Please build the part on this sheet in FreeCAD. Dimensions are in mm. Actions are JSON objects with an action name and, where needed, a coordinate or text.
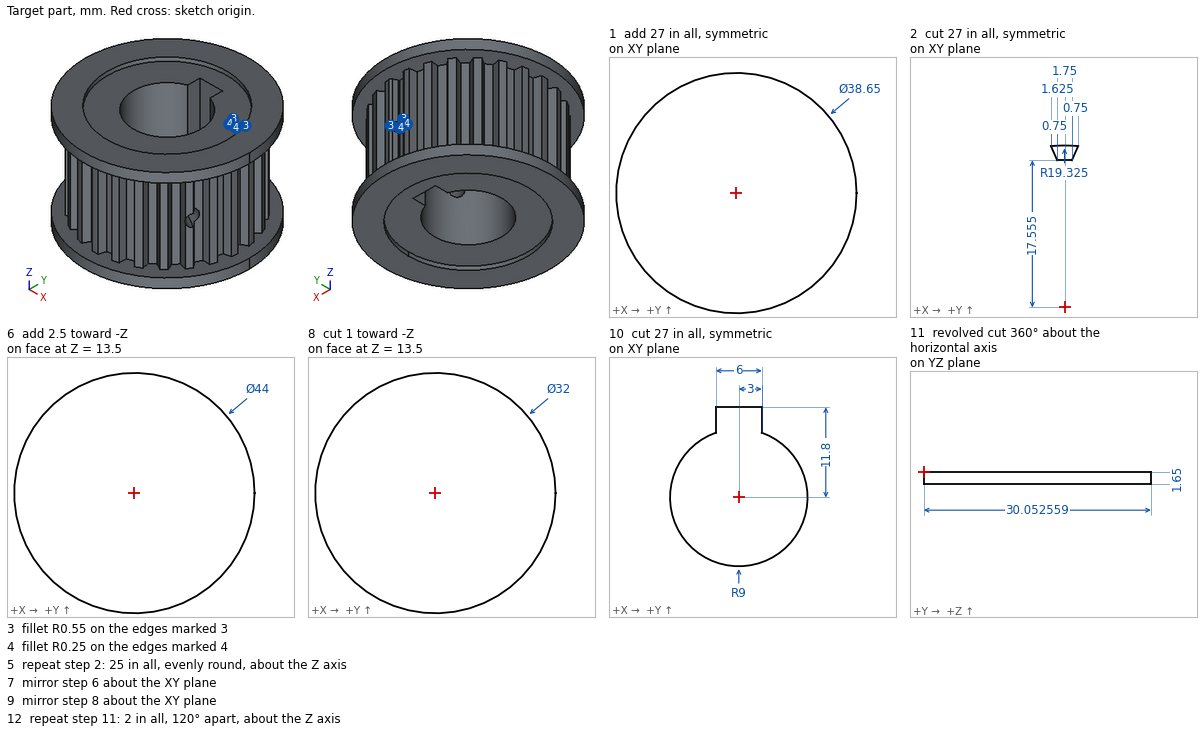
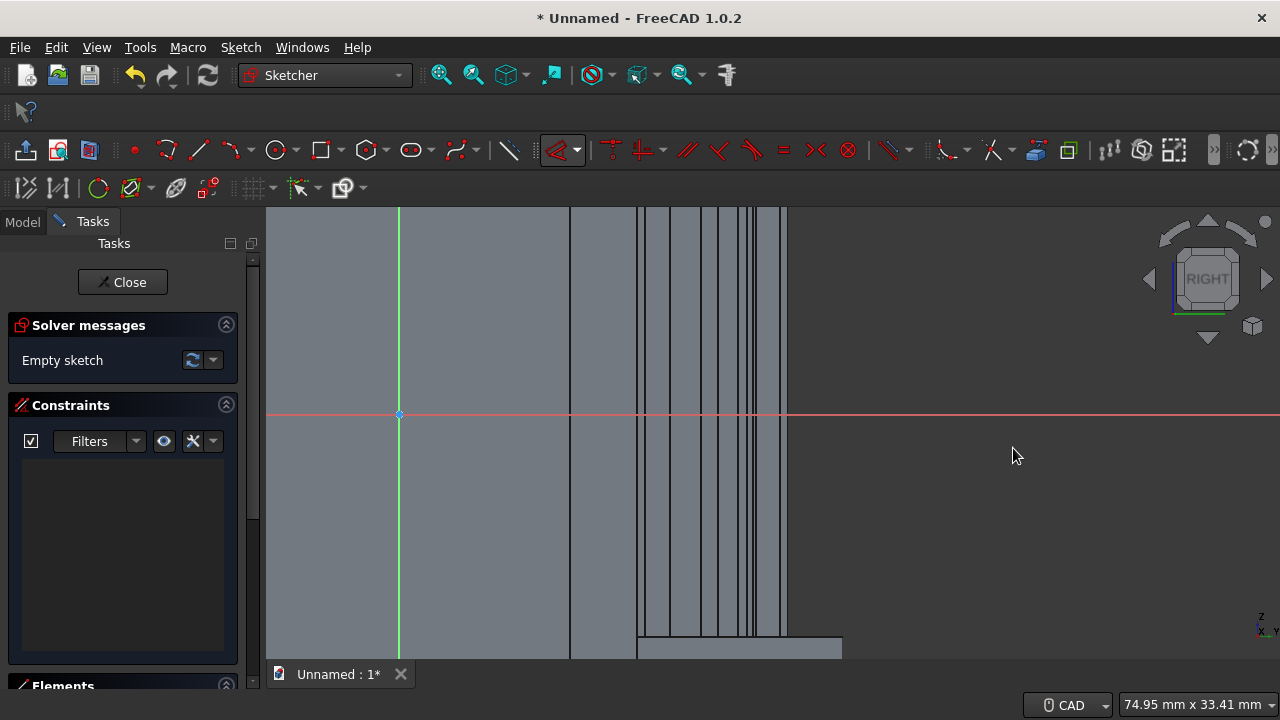
{"action": "left_click", "coordinate": [322, 150]}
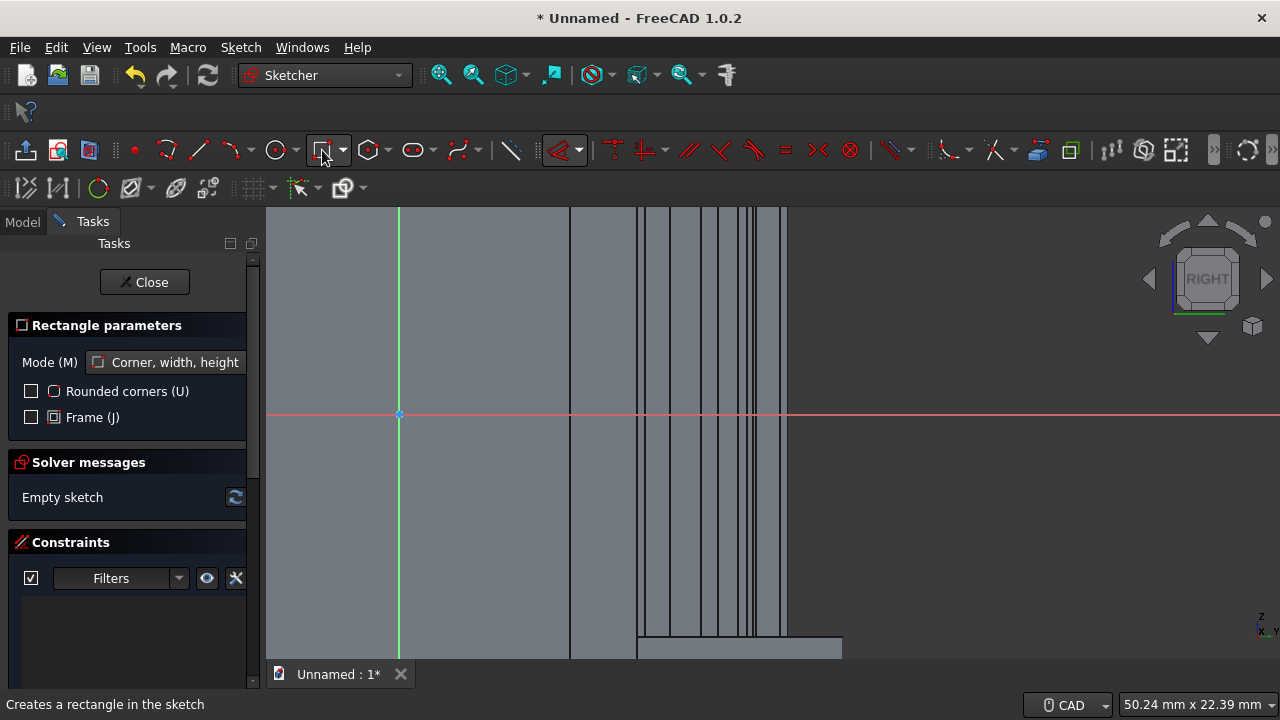
{"action": "left_click", "coordinate": [399, 415]}
{"action": "mouse_move", "coordinate": [1006, 448]}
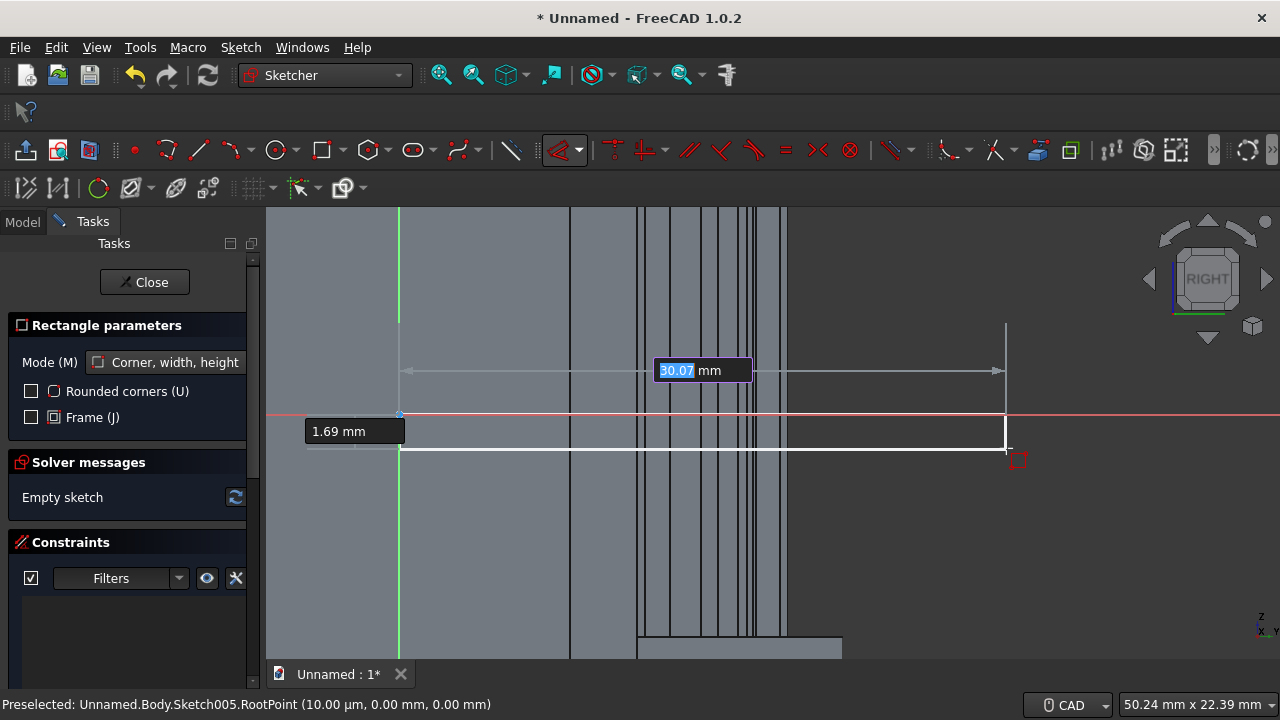
{"action": "type", "text": "30.052559"}
{"action": "key", "text": "Tab"}
{"action": "type", "text": "1.65"}
{"action": "key", "text": "Return"}
{"action": "key", "text": "Escape"}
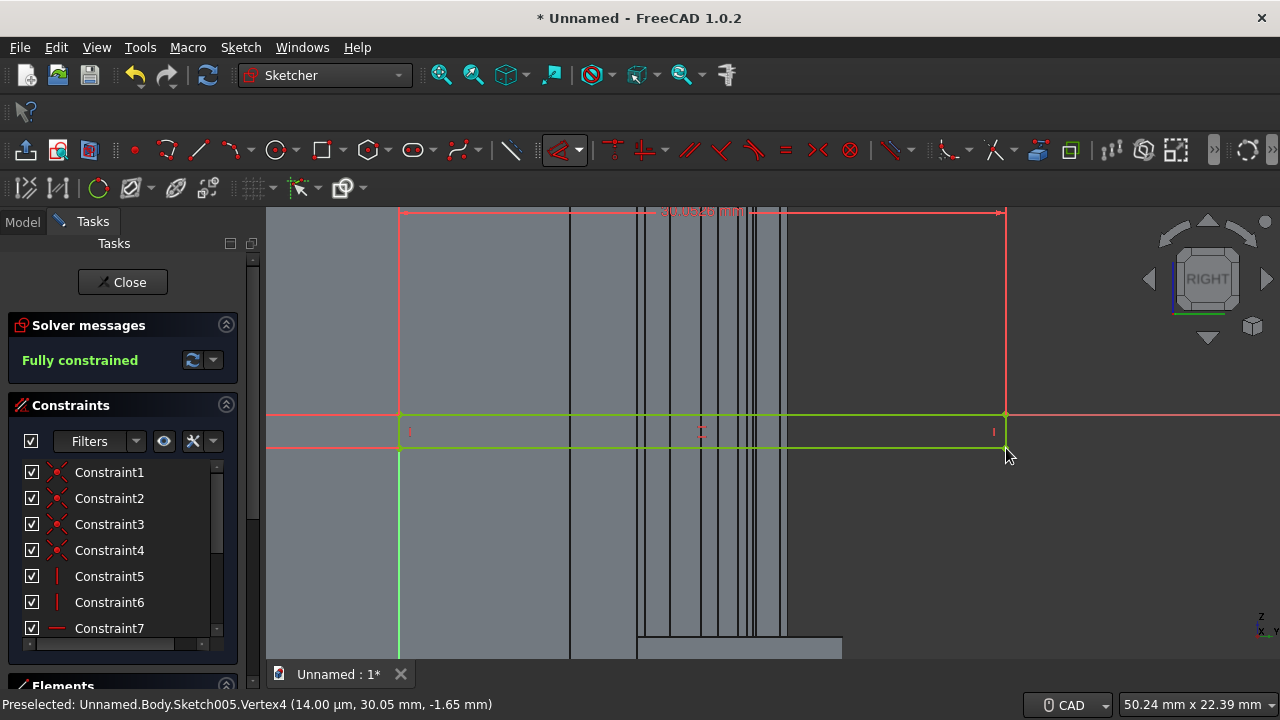
{"action": "left_click", "coordinate": [123, 282]}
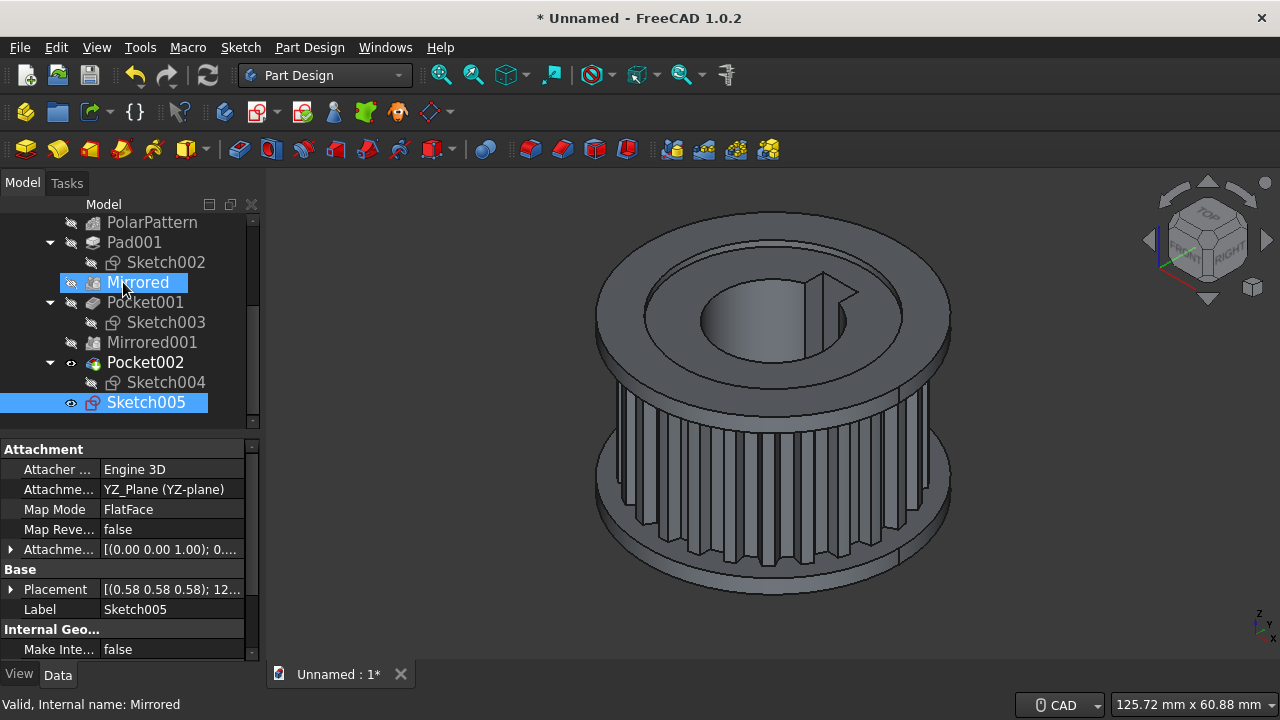
{"action": "left_click", "coordinate": [304, 150]}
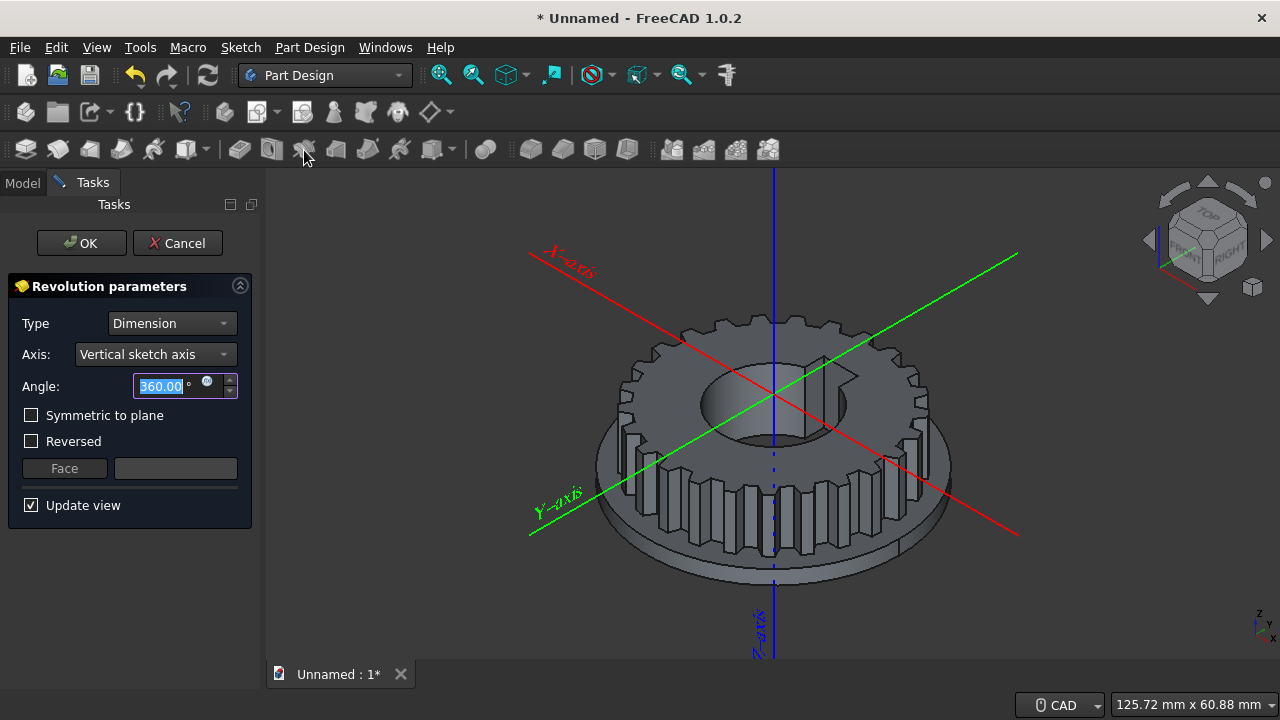
{"action": "left_click", "coordinate": [156, 354]}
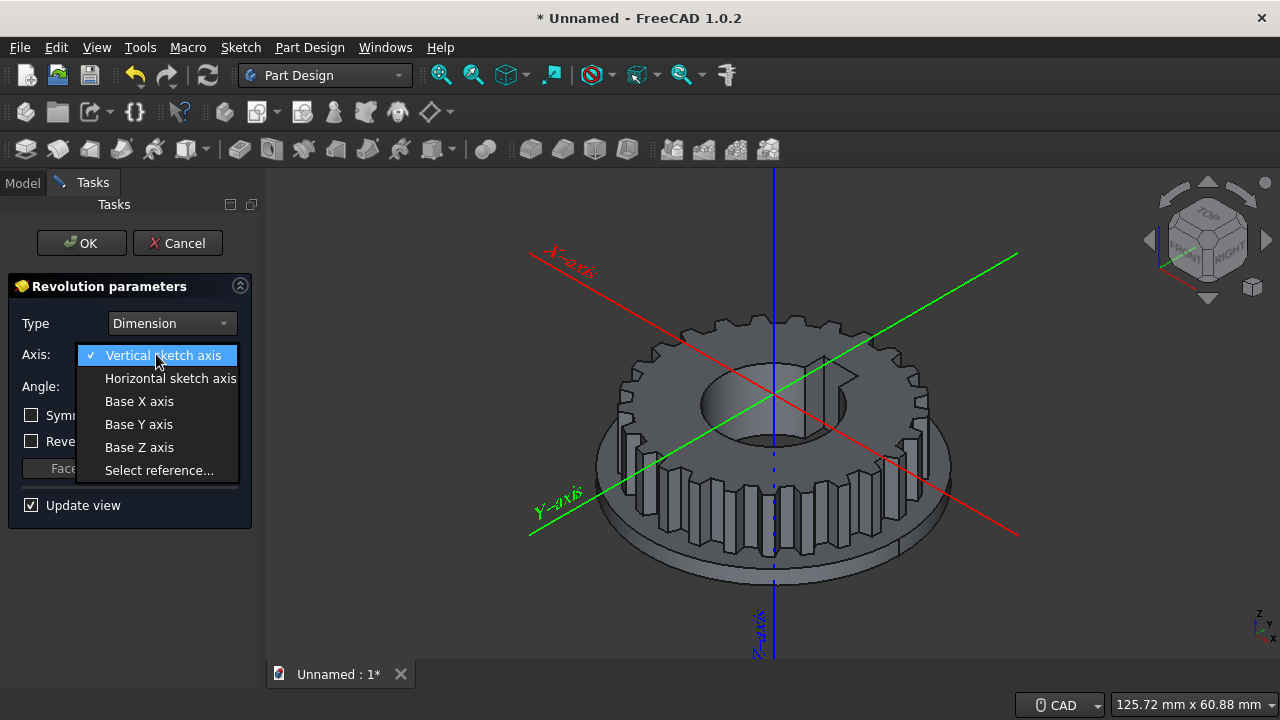
{"action": "left_click", "coordinate": [156, 378]}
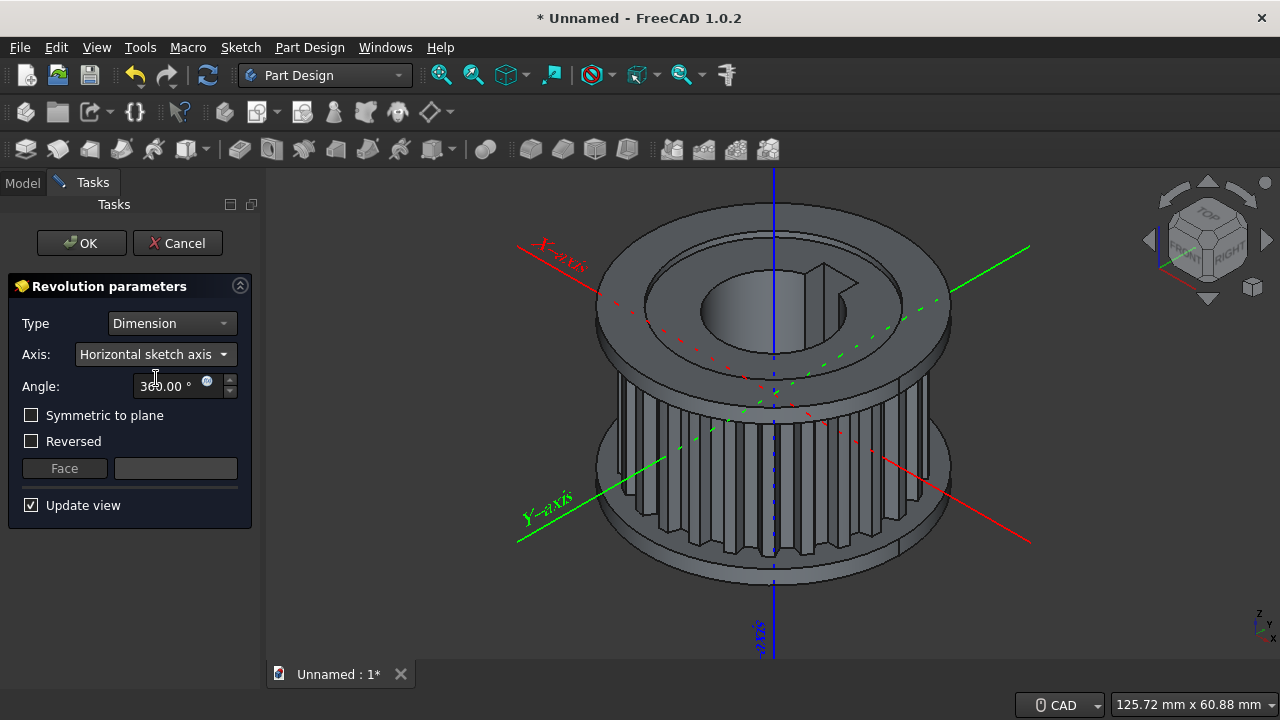
{"action": "left_click", "coordinate": [82, 243]}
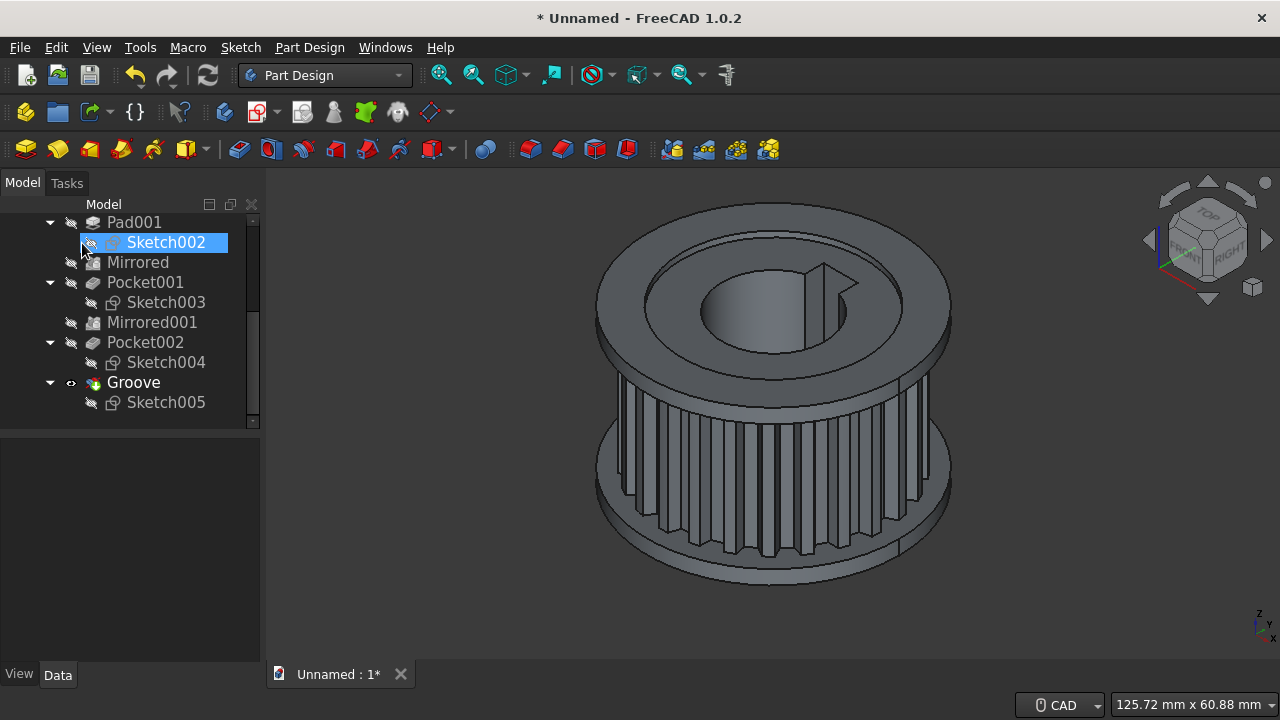
{"action": "left_click", "coordinate": [442, 76]}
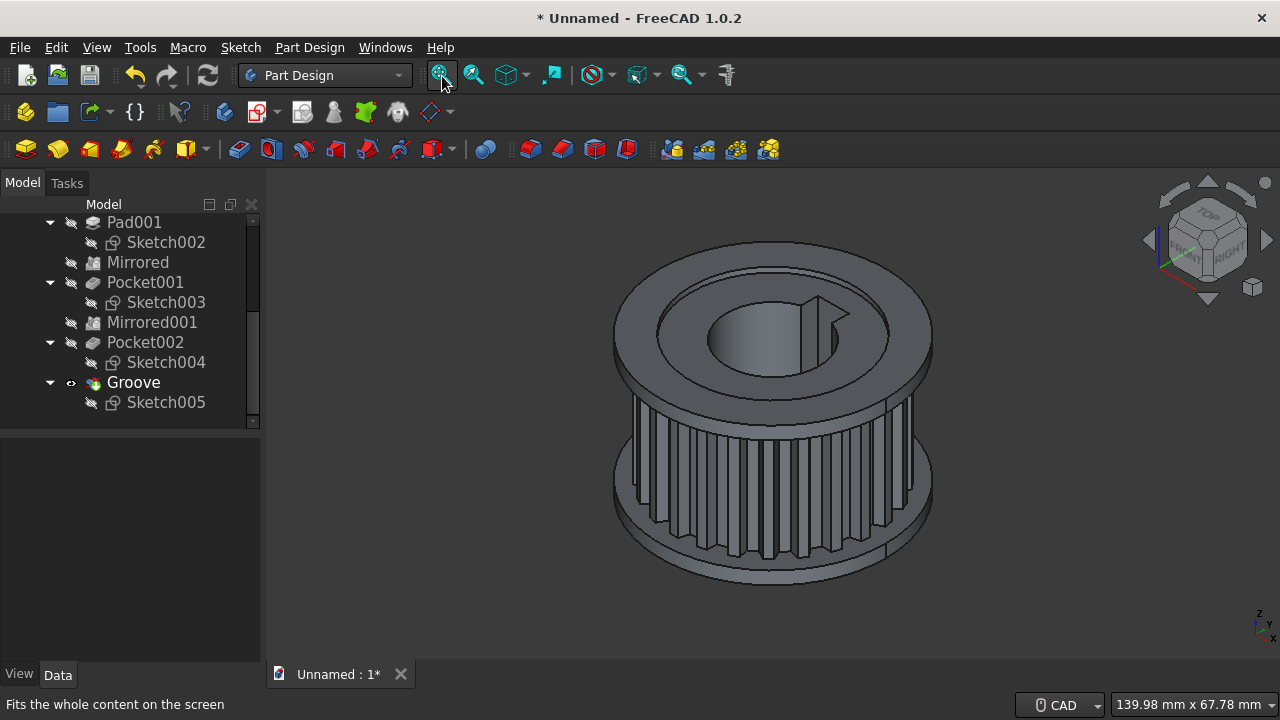
{"action": "left_click", "coordinate": [116, 383]}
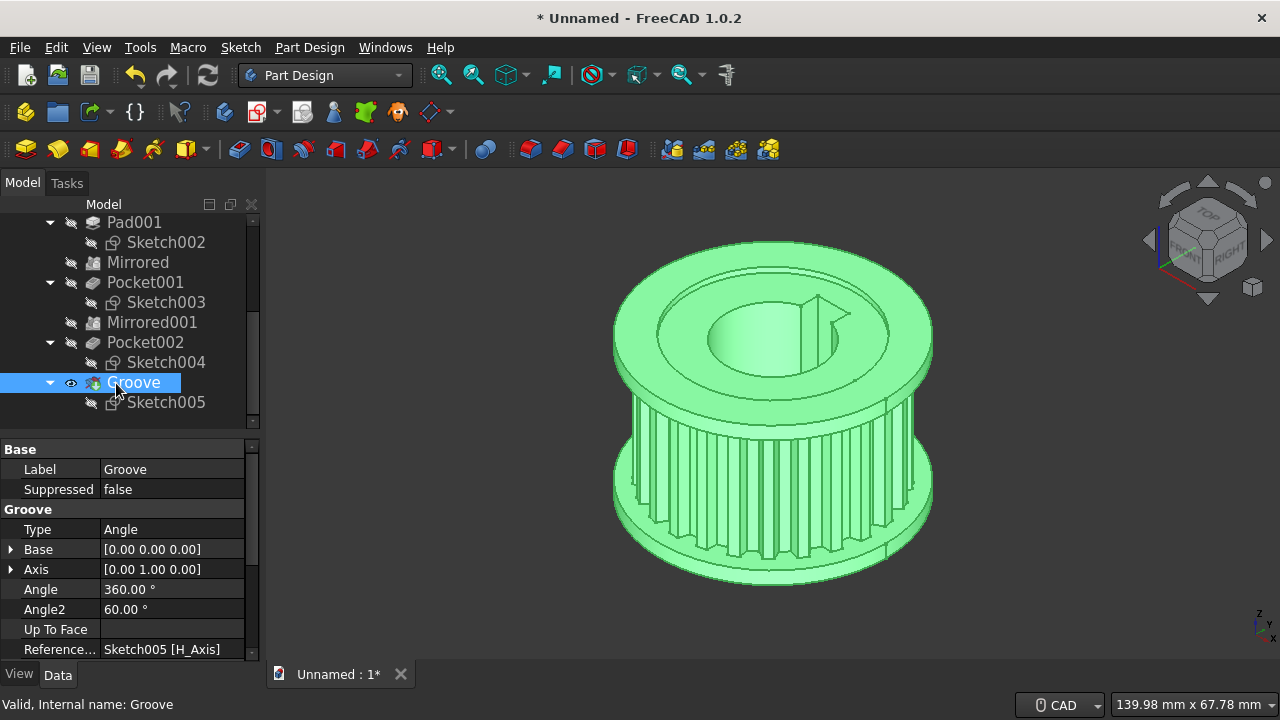
{"action": "left_click", "coordinate": [736, 150]}